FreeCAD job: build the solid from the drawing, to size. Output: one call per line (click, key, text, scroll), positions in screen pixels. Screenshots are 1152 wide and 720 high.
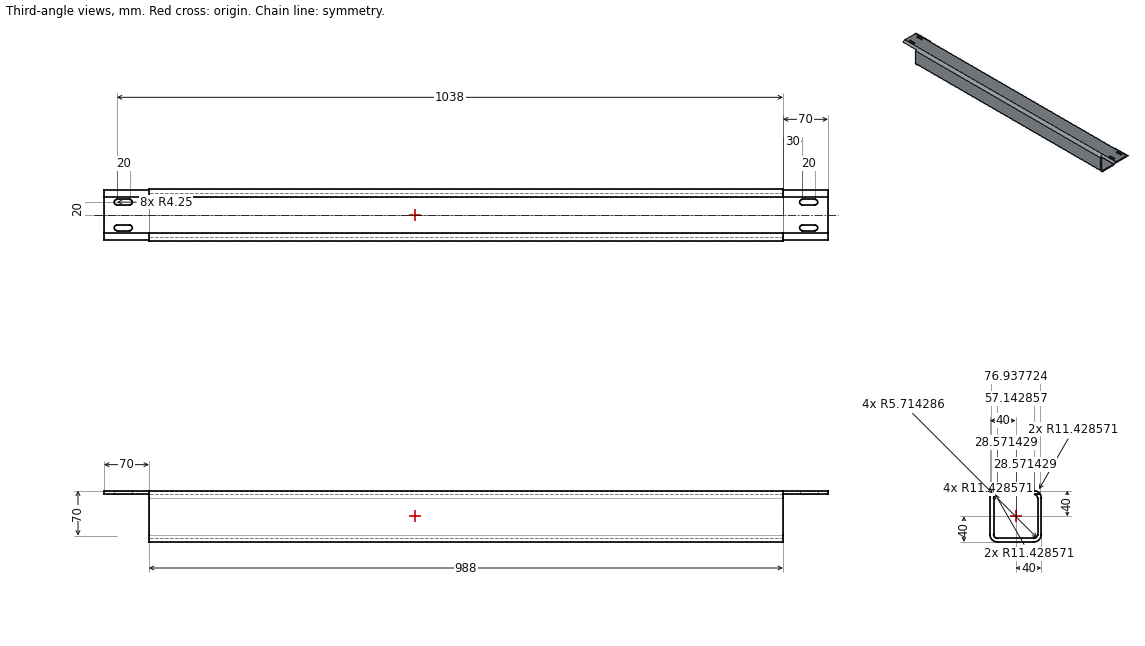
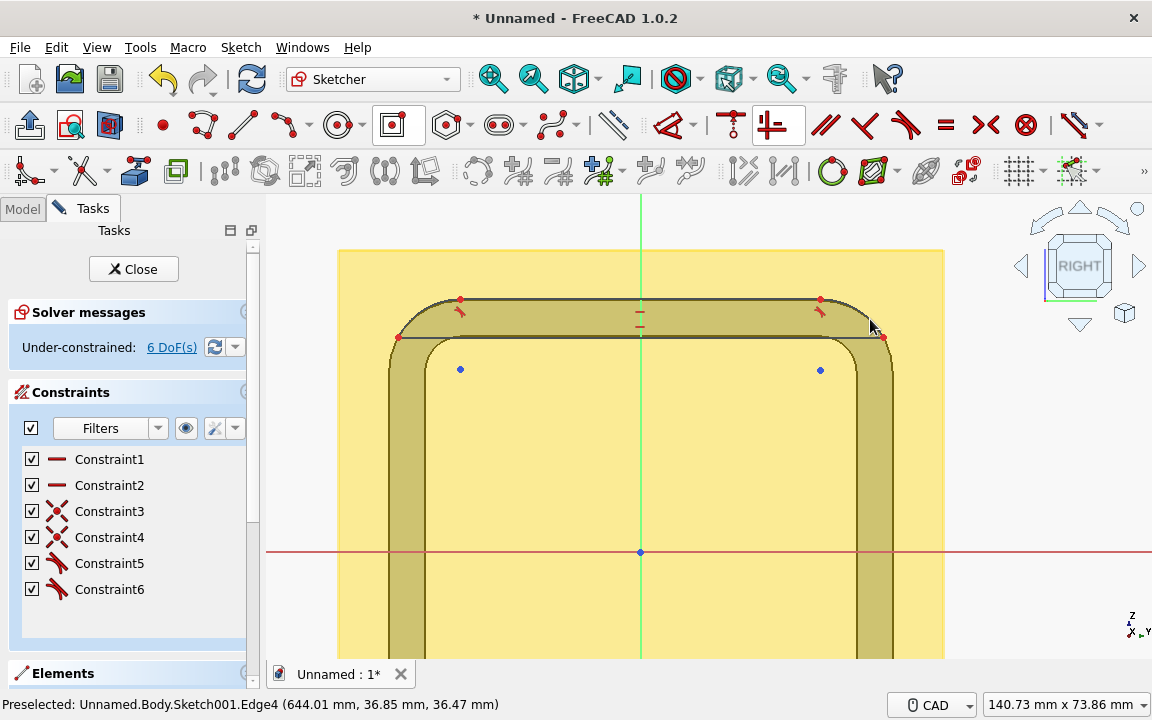
click(438, 303)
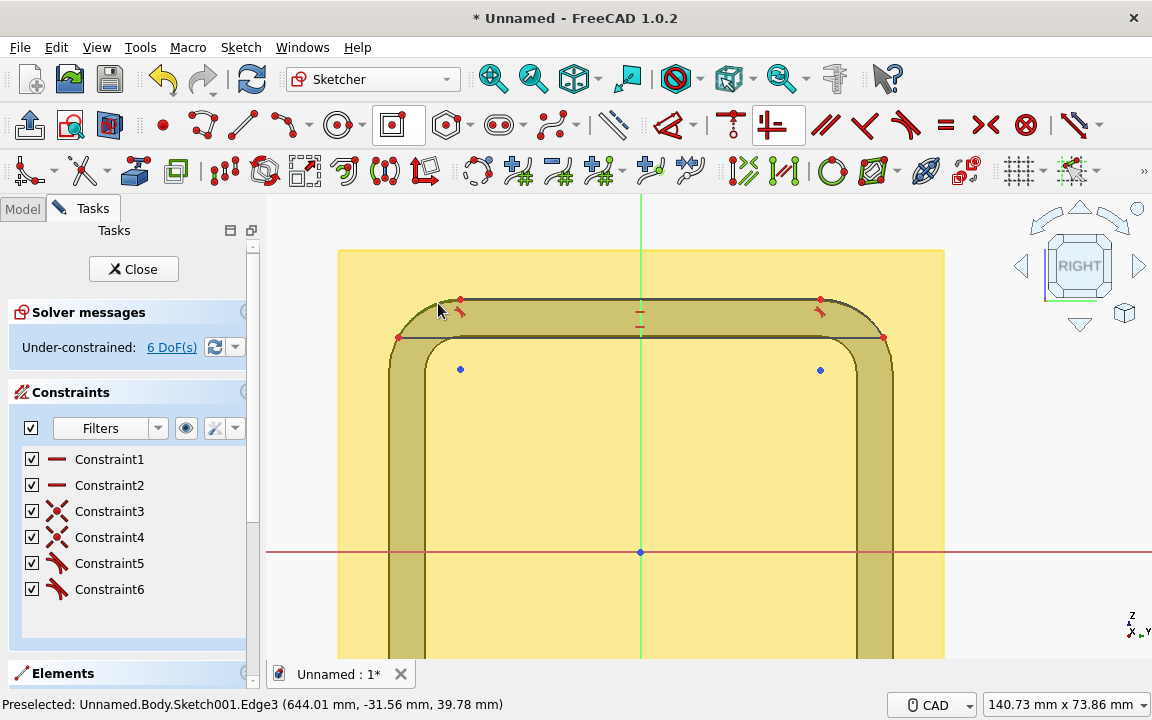
click(870, 319)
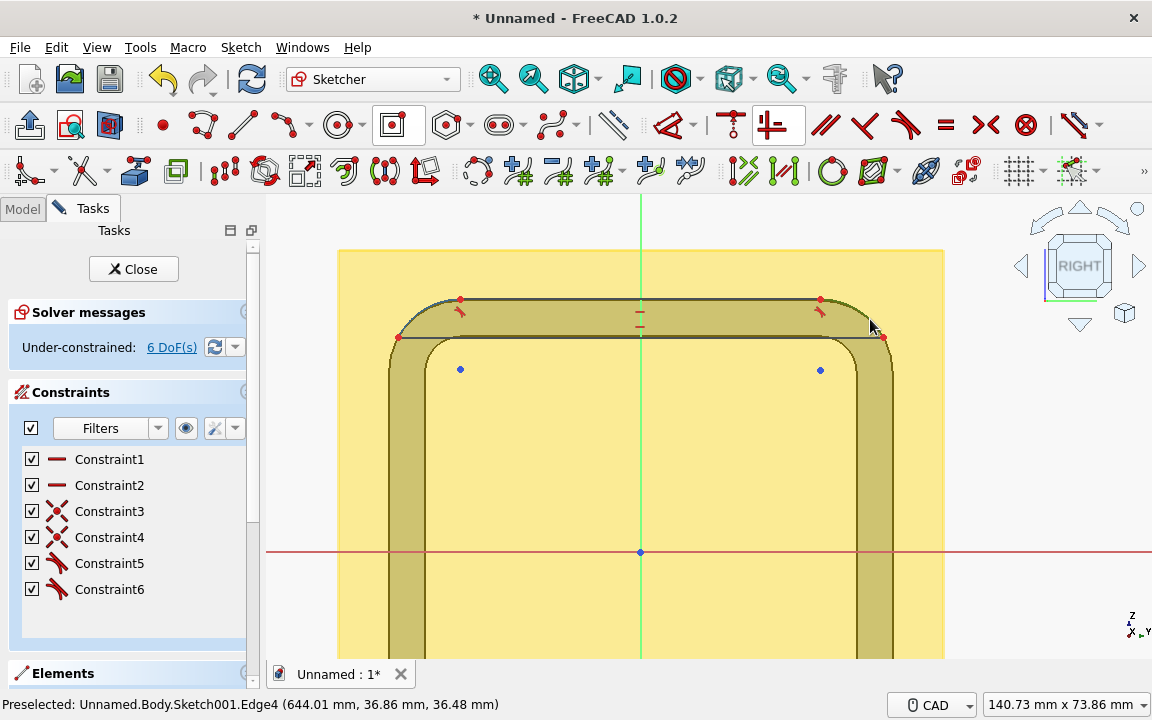
key(e)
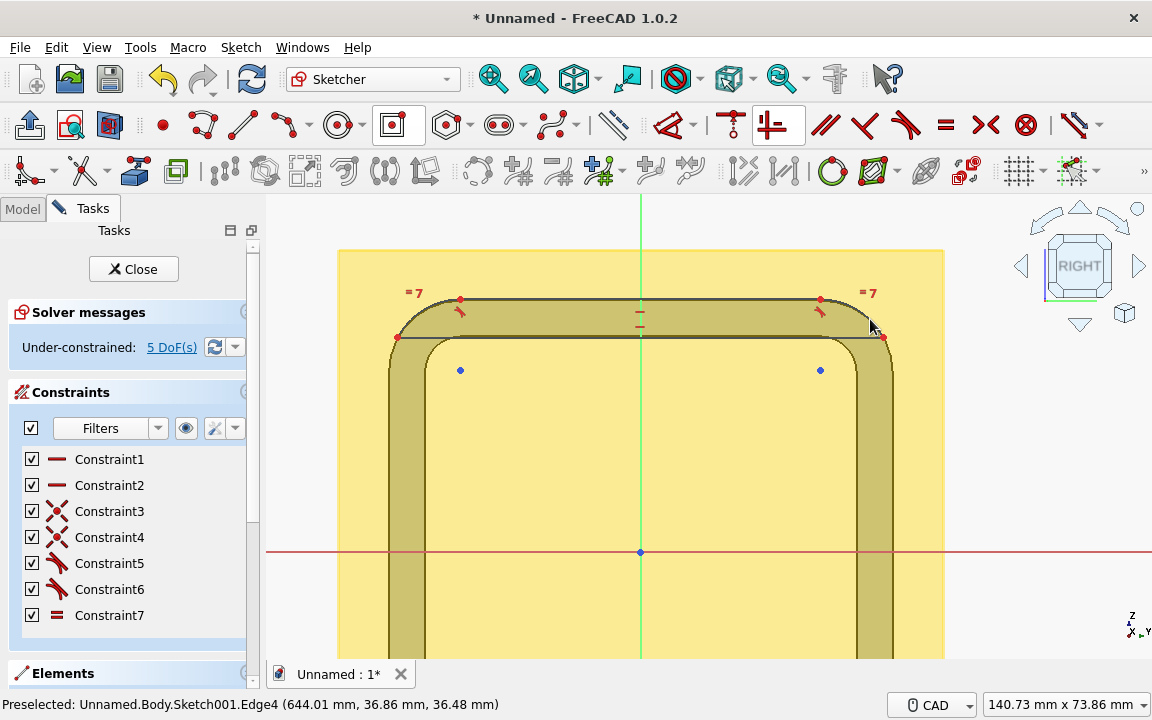
key(d)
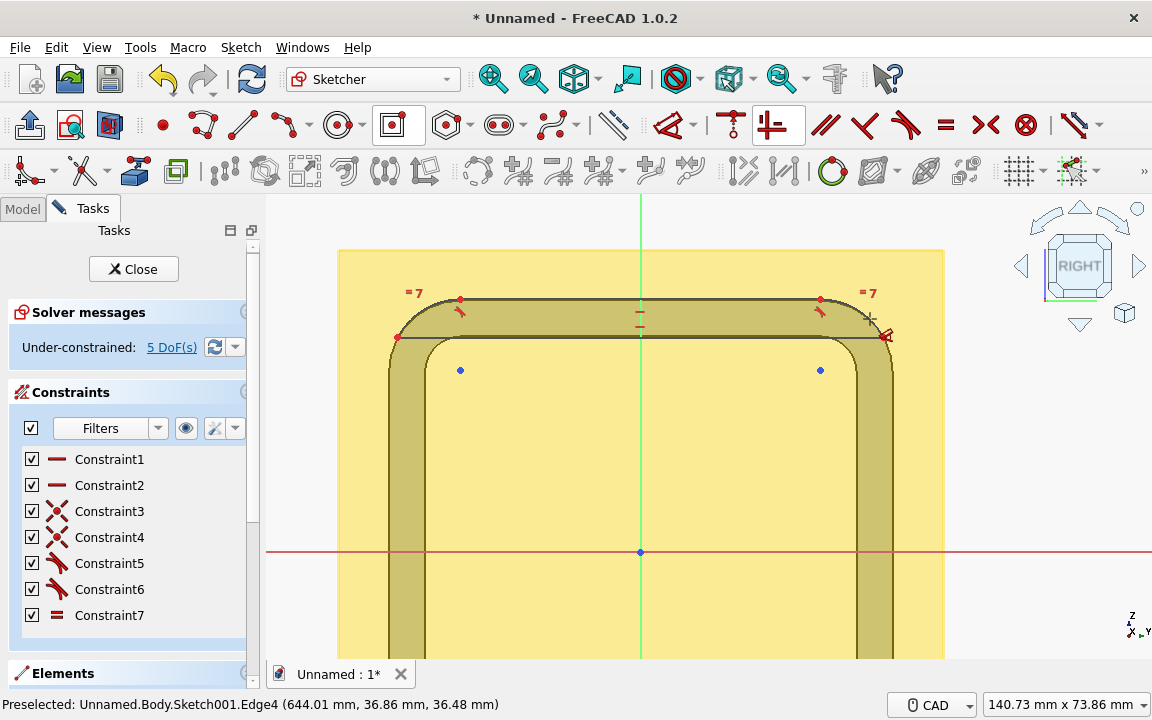
click(438, 303)
click(428, 273)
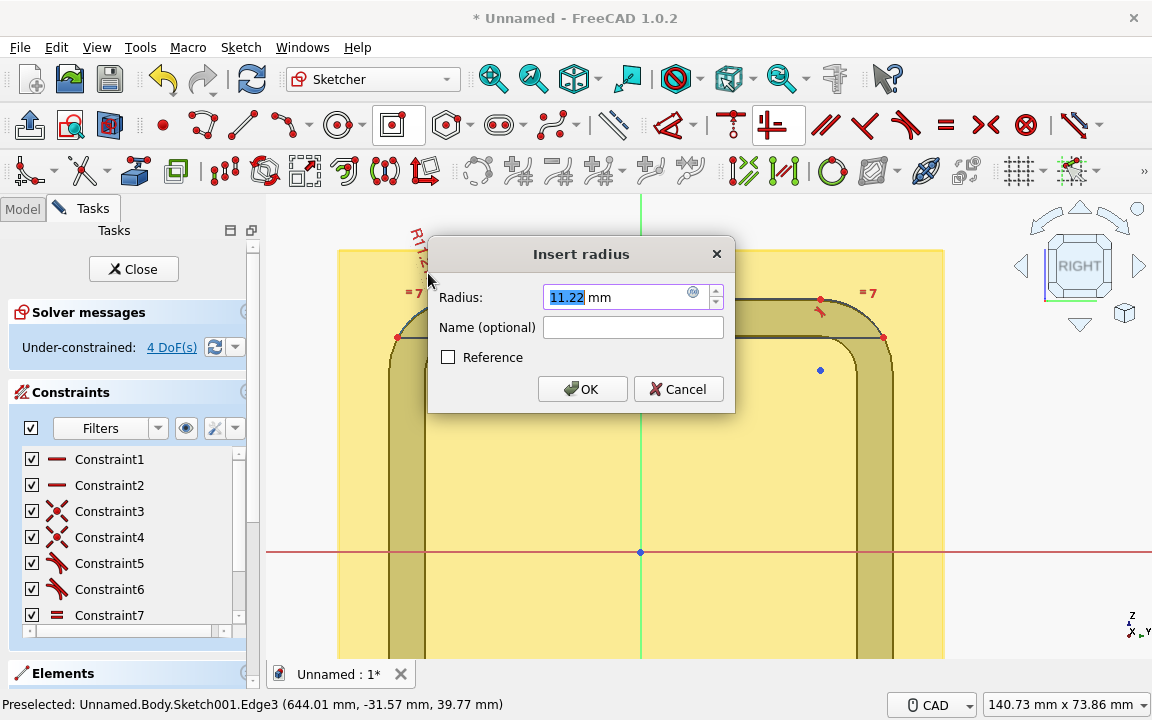
text(11.428571)
key(Return)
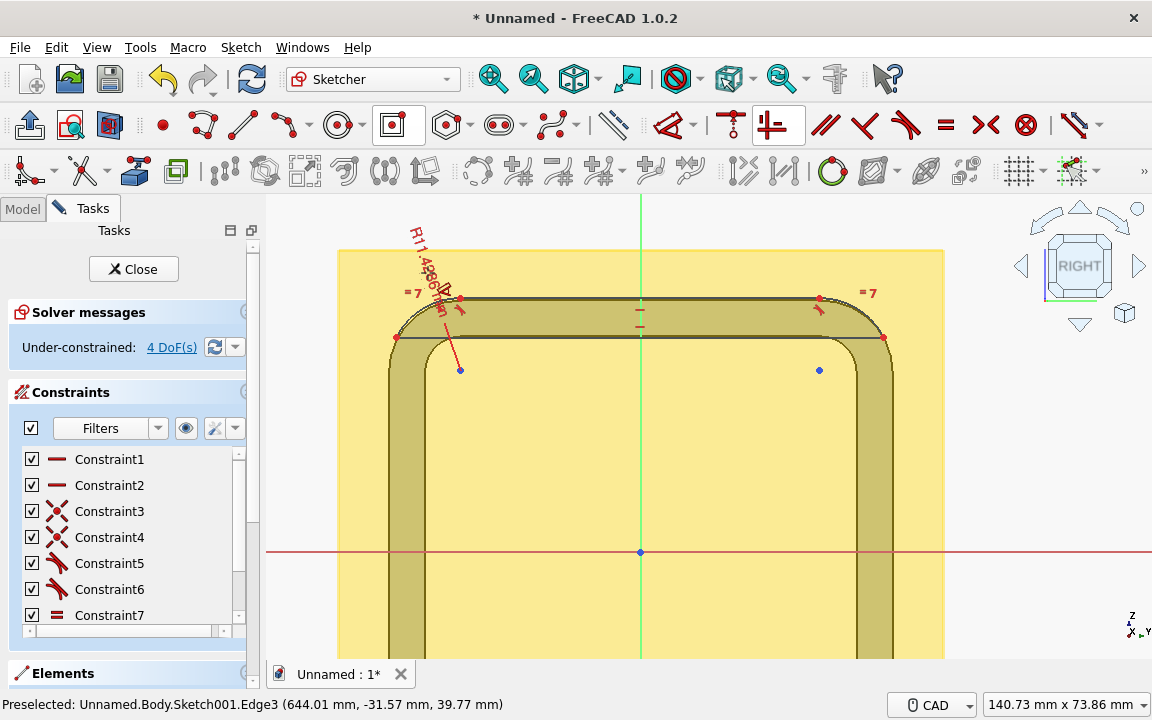
click(820, 298)
click(854, 425)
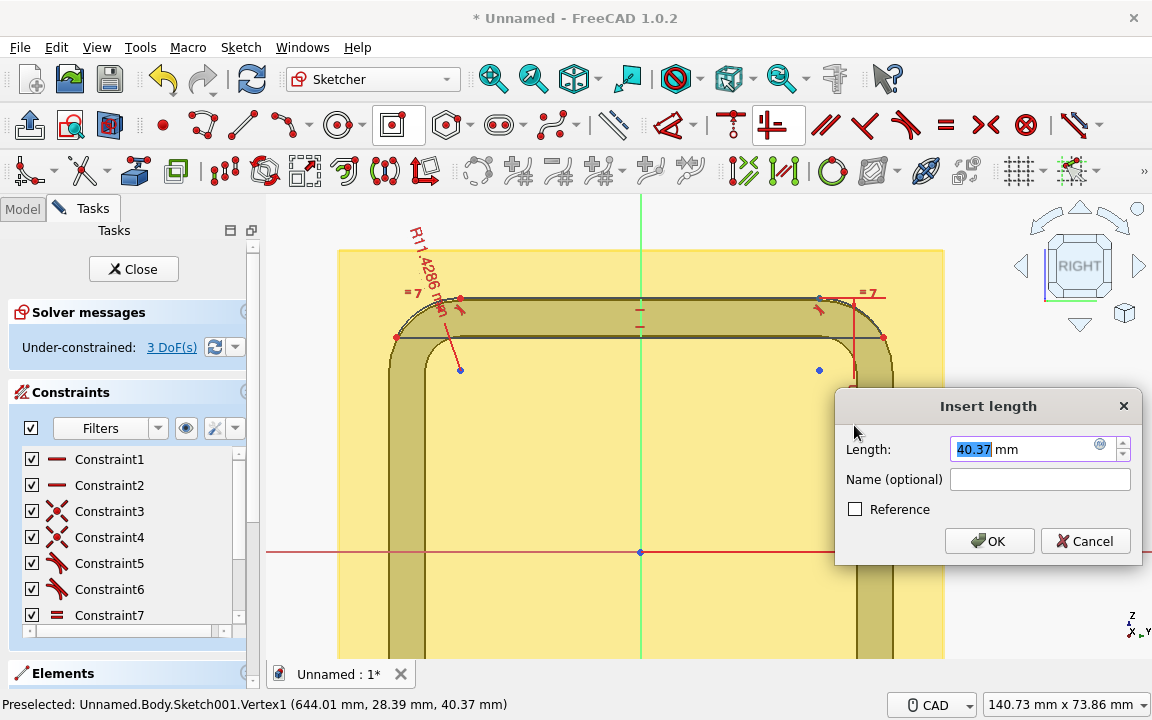
text(40)
key(Return)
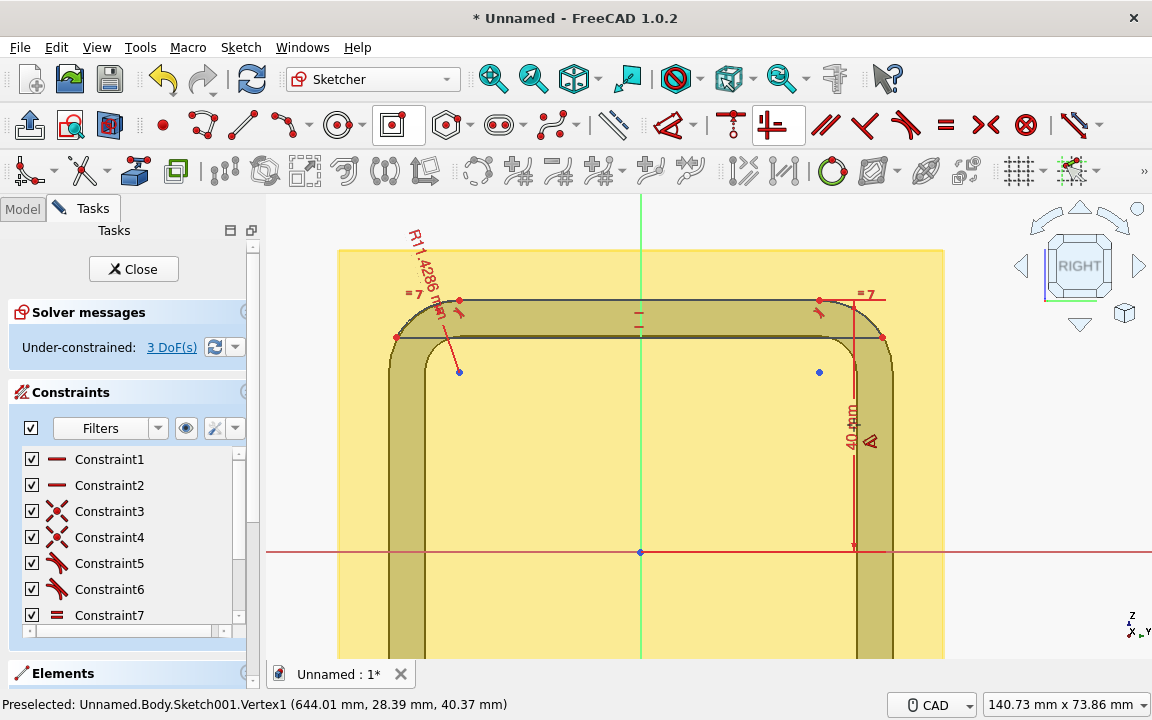
click(711, 300)
click(557, 266)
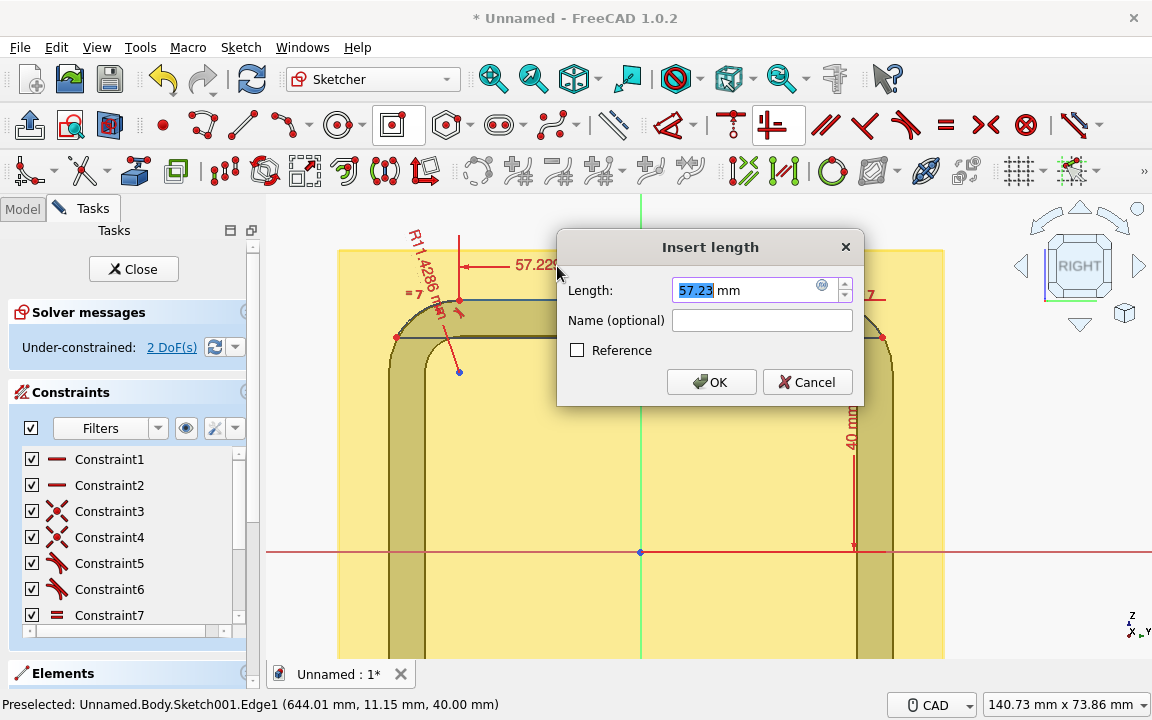
text(57.142857)
key(Return)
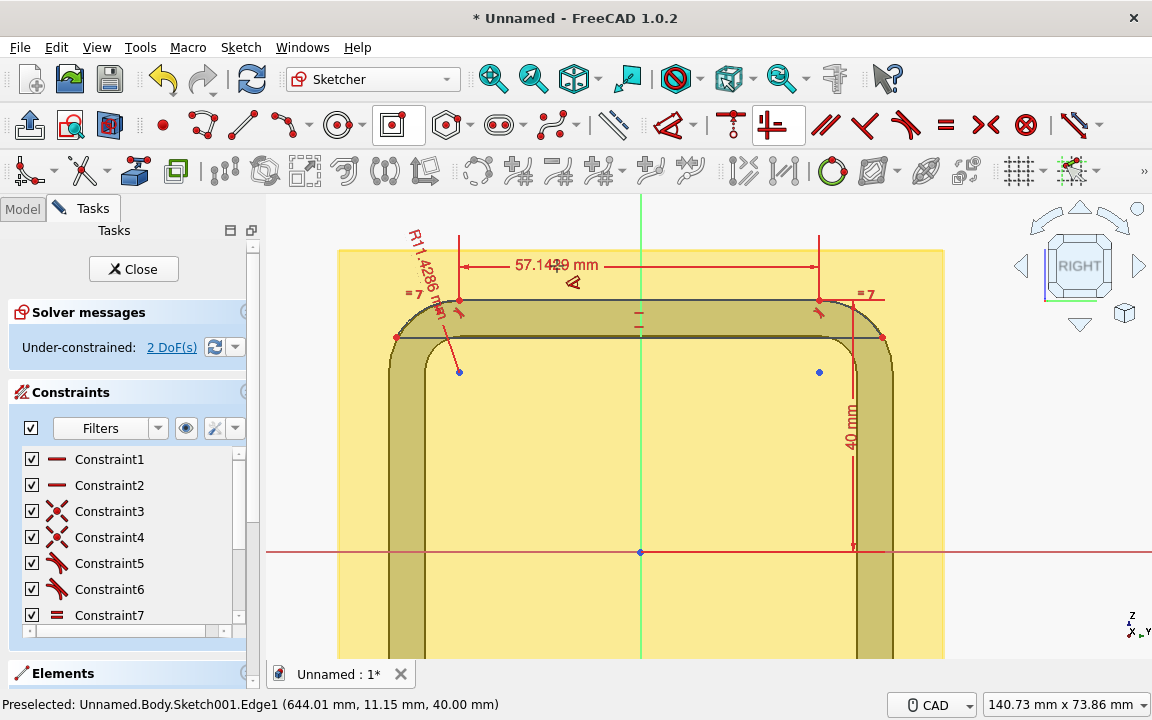
click(542, 338)
click(527, 372)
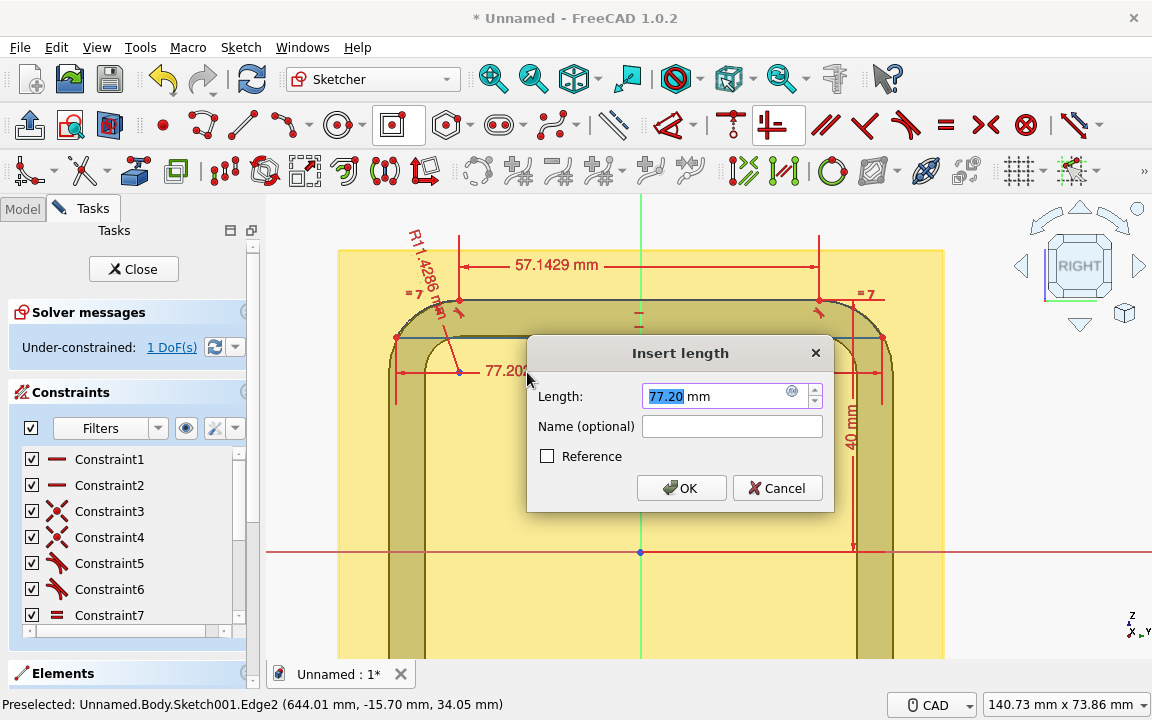
text(76.937724)
key(Return)